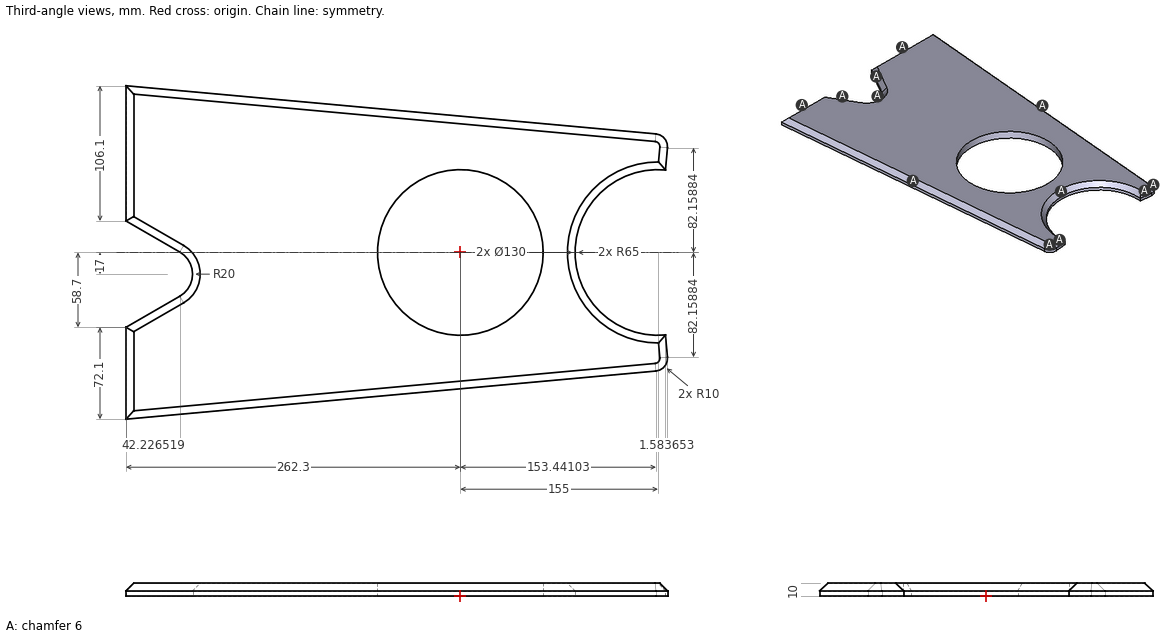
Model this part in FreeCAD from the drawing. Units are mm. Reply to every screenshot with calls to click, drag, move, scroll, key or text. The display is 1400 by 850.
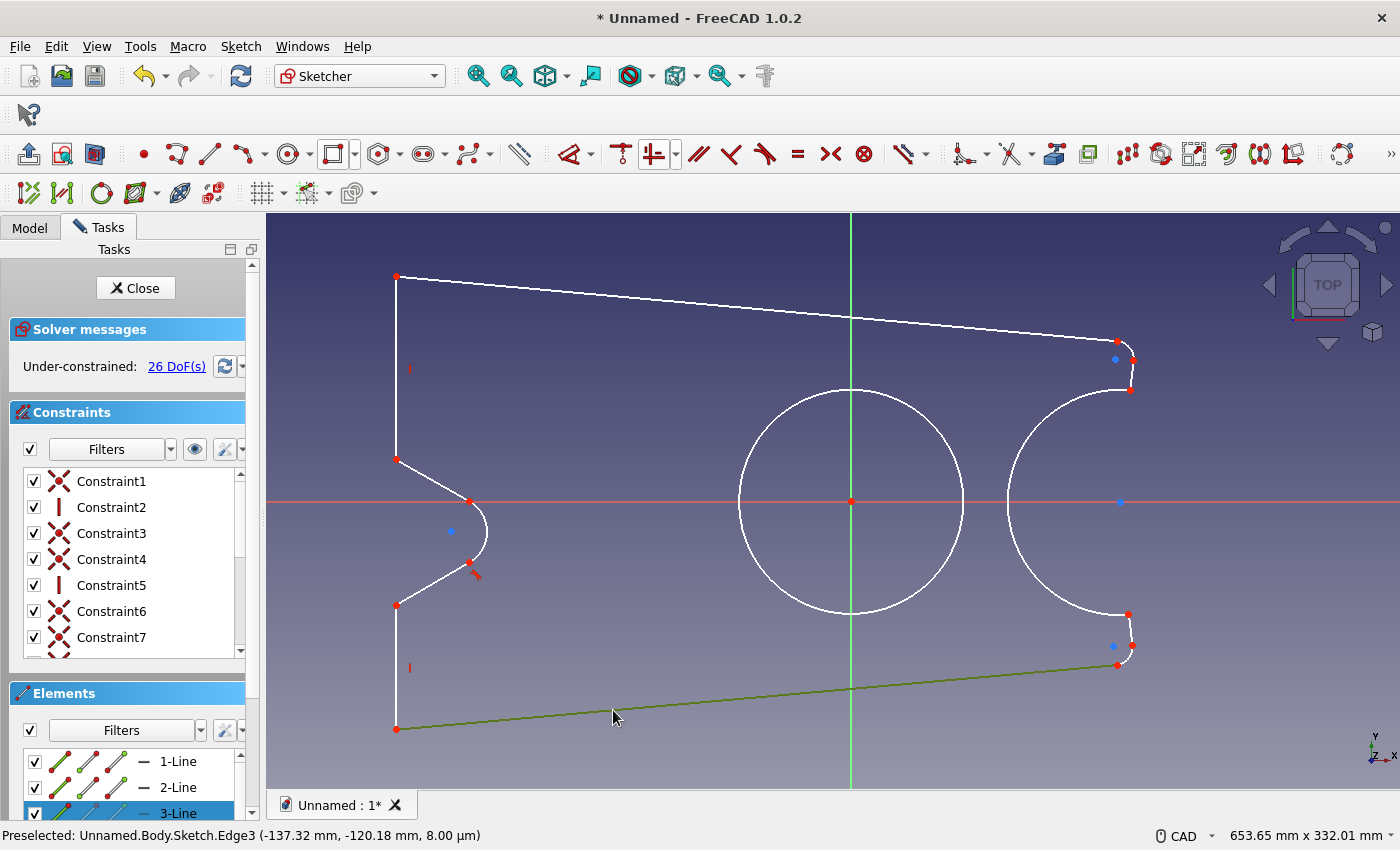
click(1129, 658)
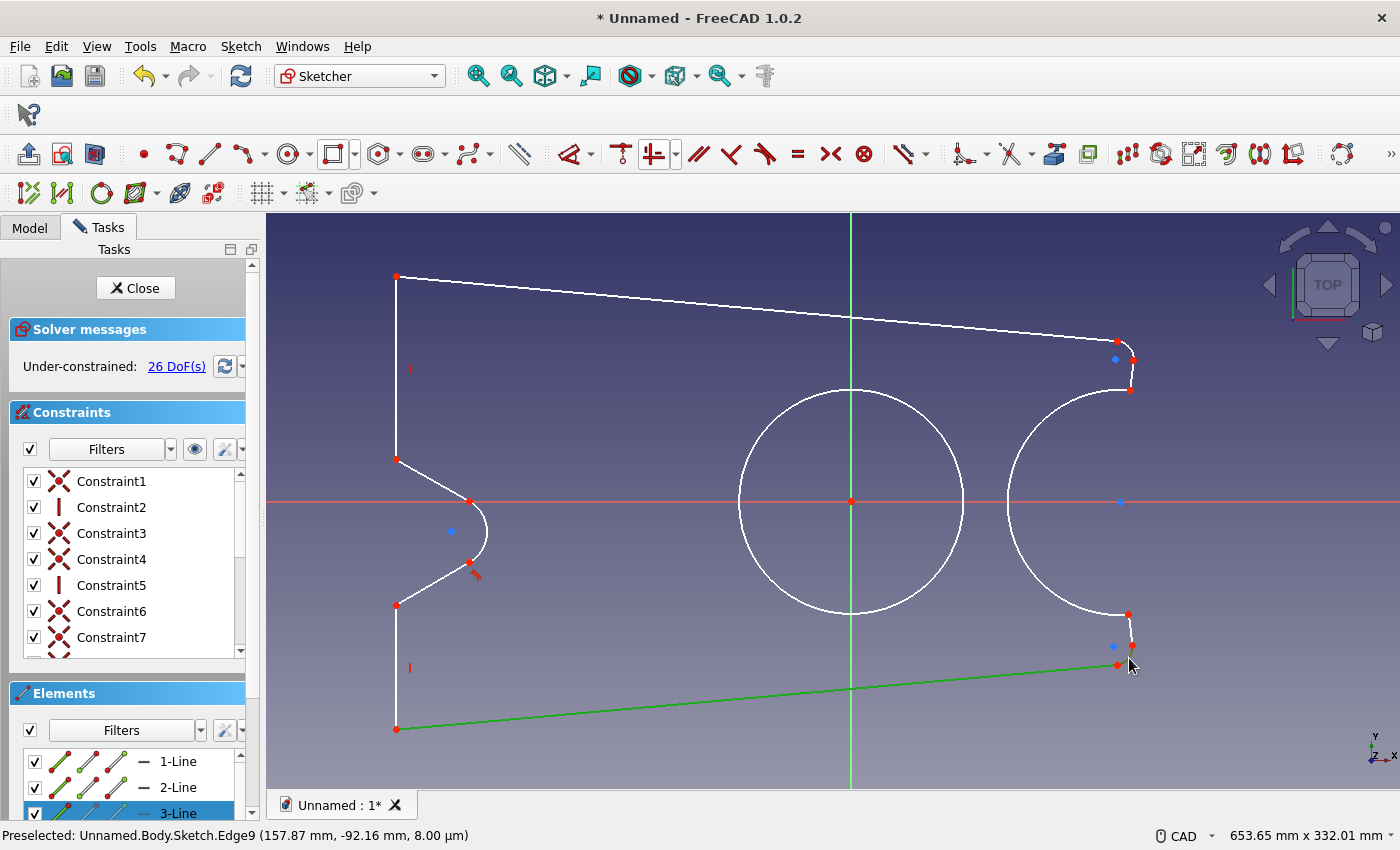
click(765, 154)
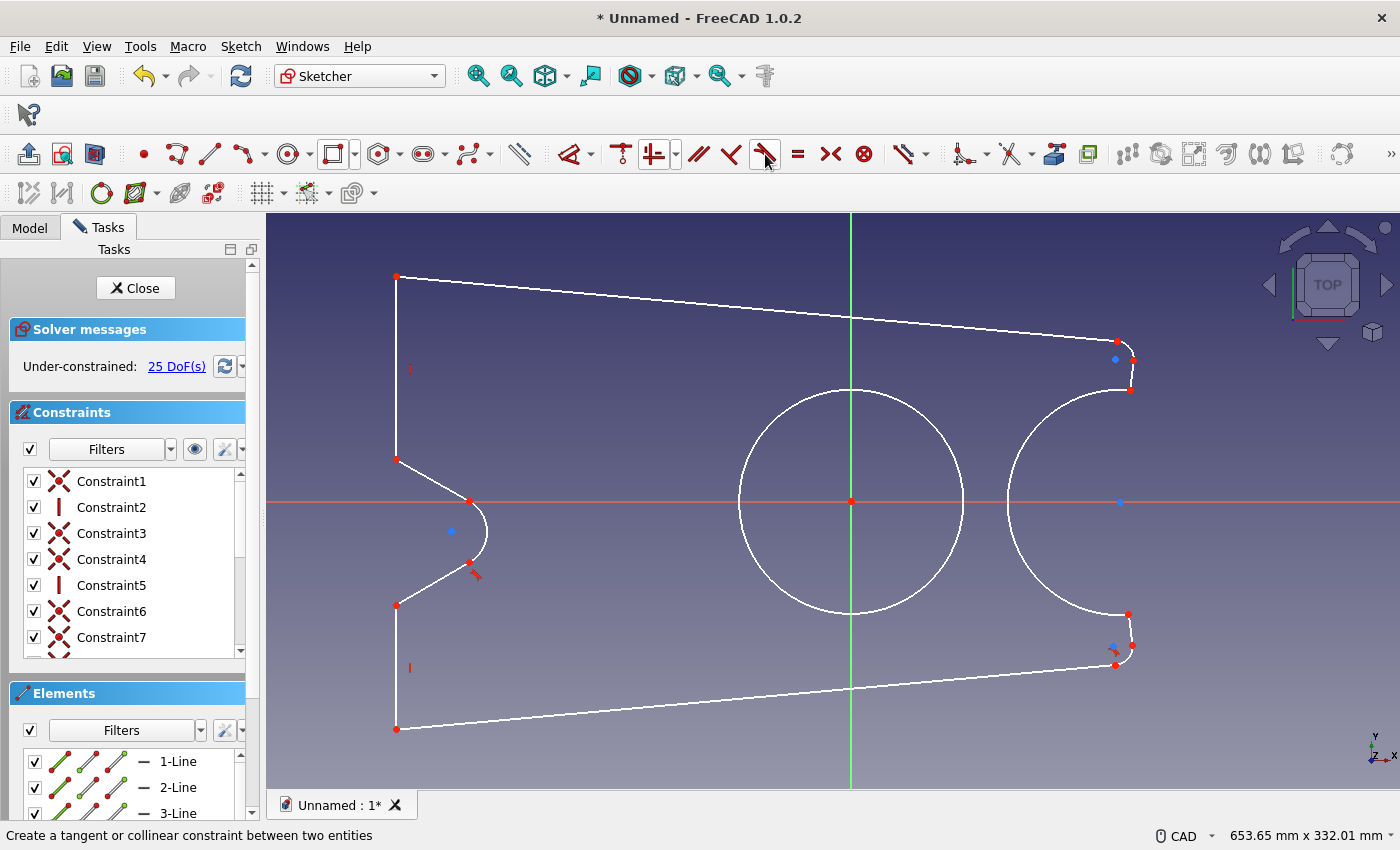
scroll(1131, 636, up, 3)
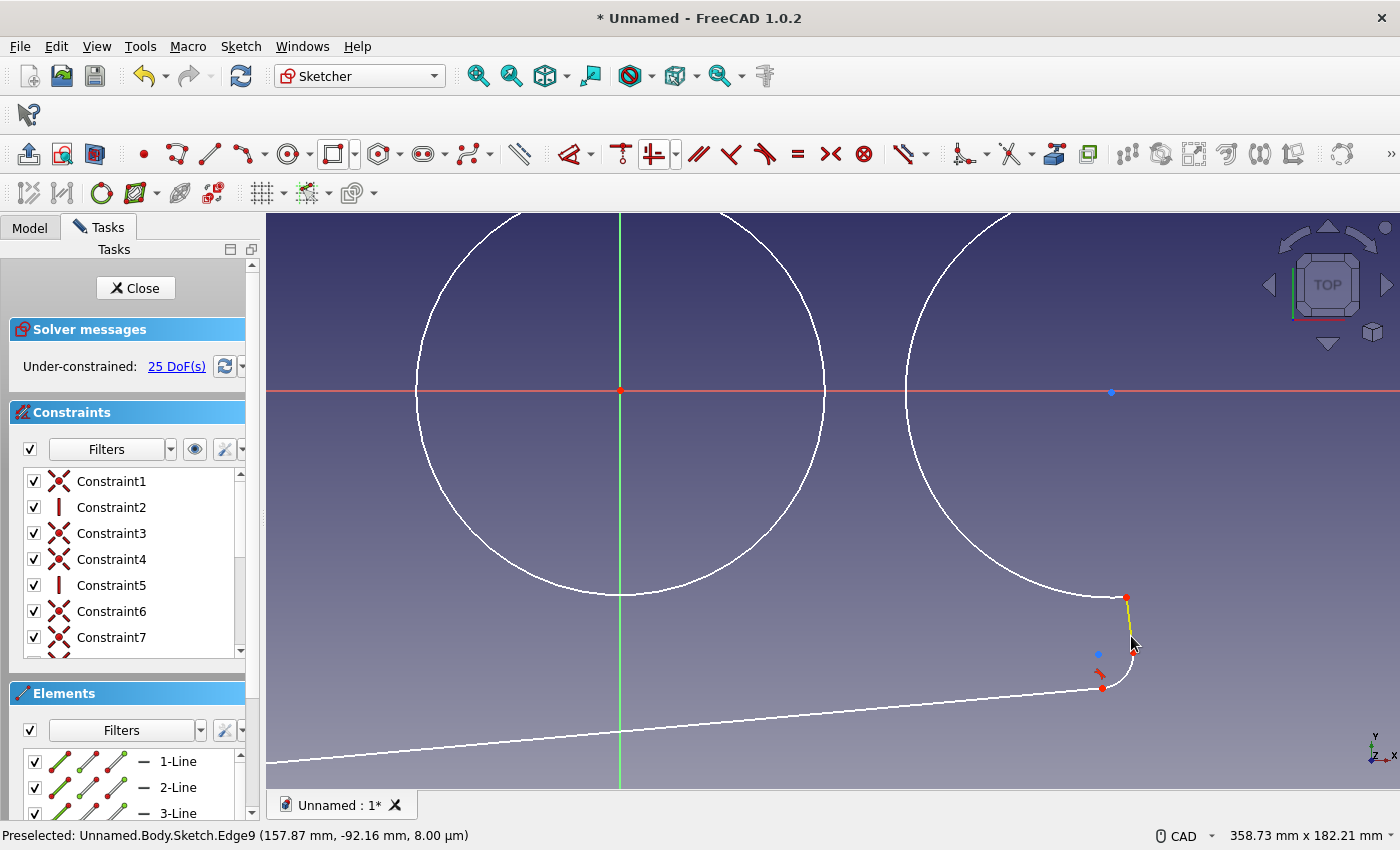
click(1131, 636)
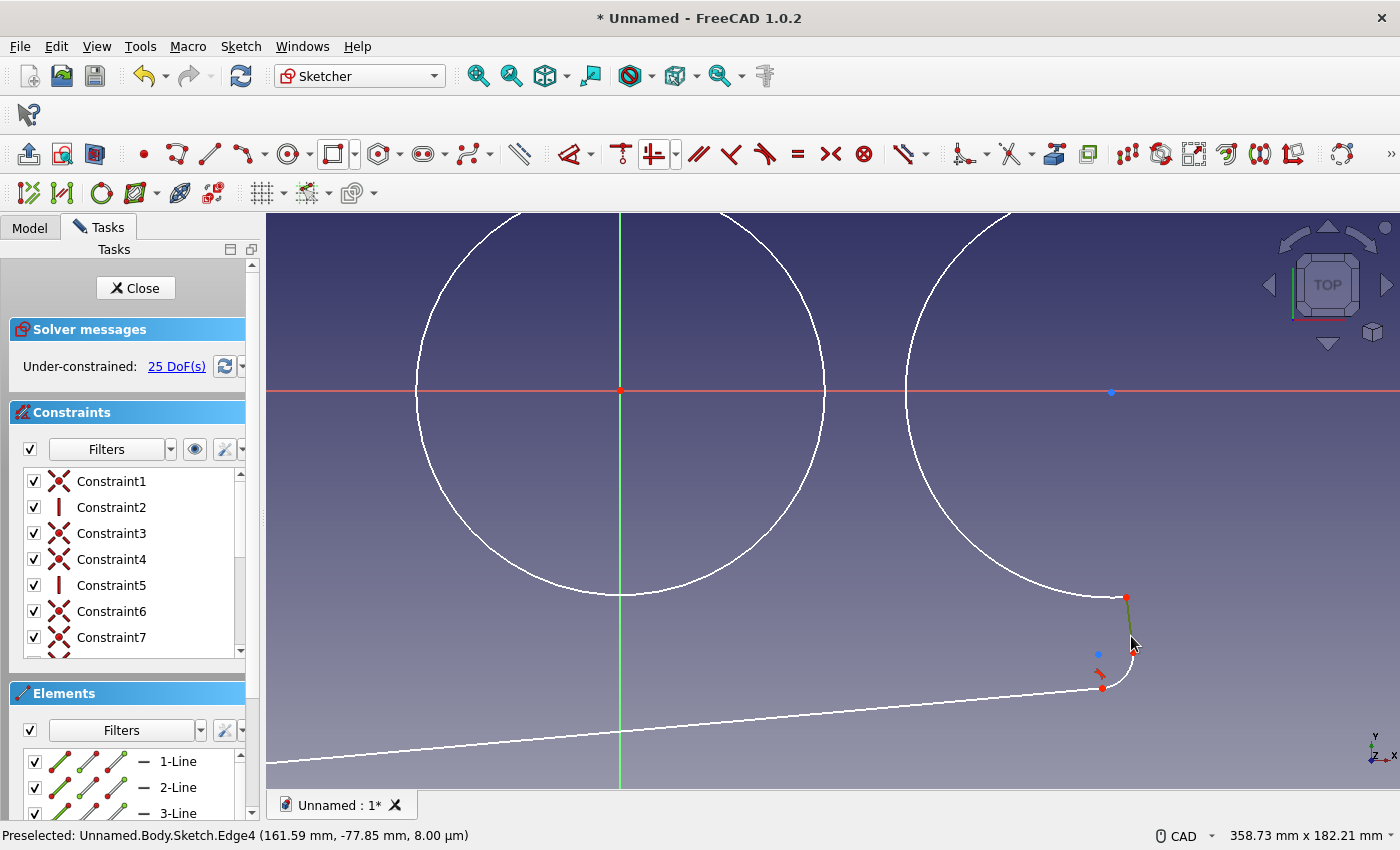
click(1117, 683)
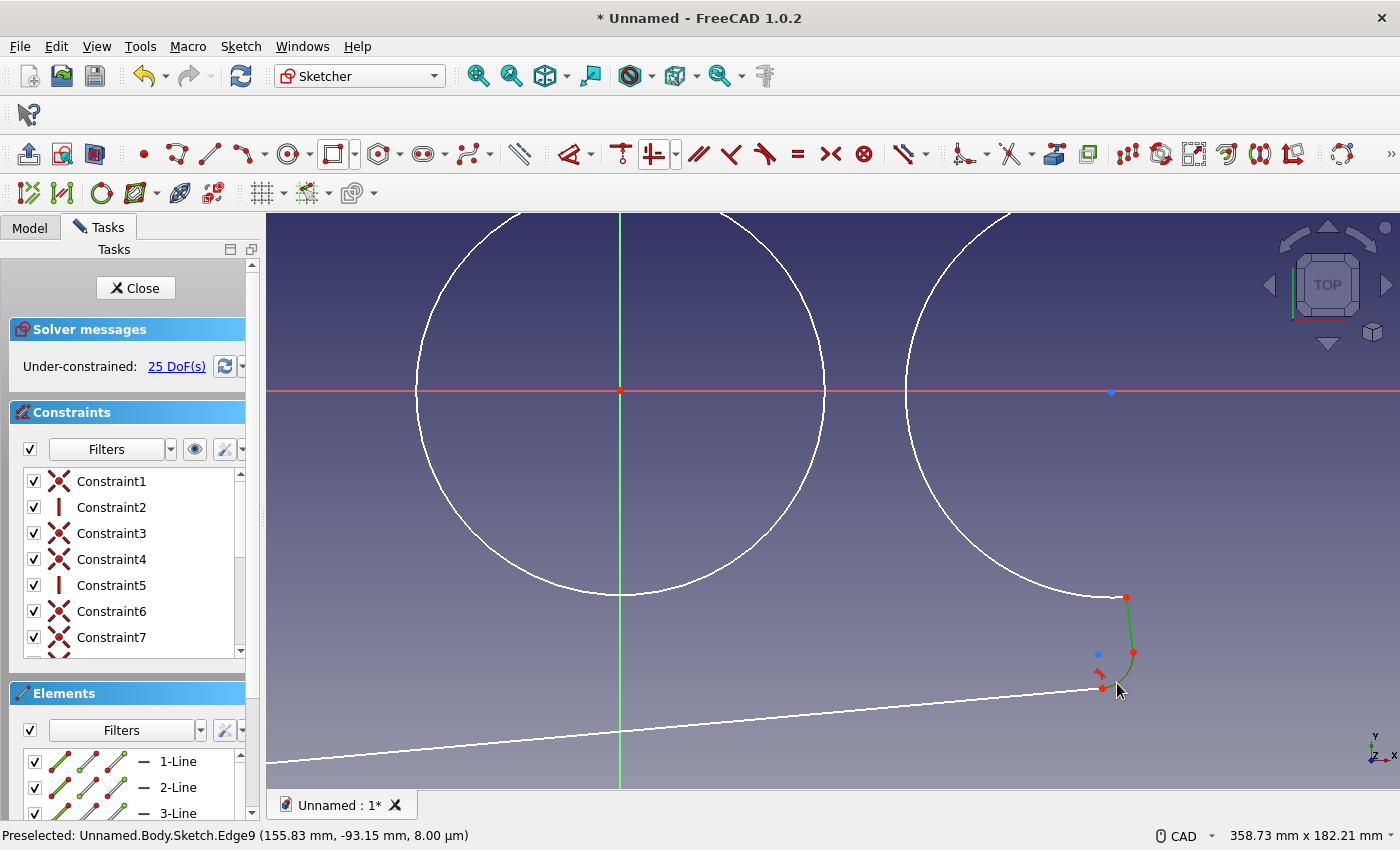
click(765, 154)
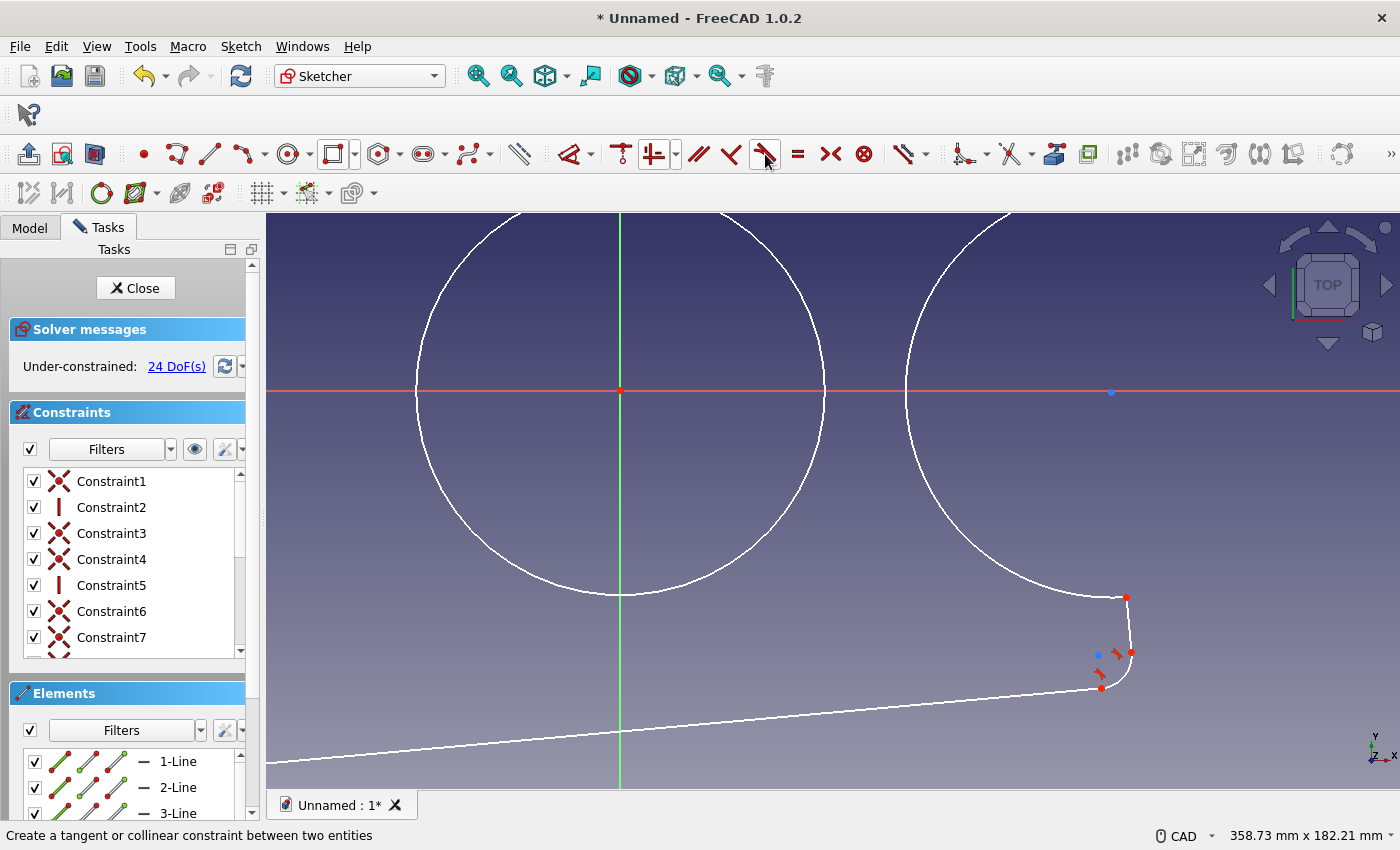
scroll(1011, 591, down, 4)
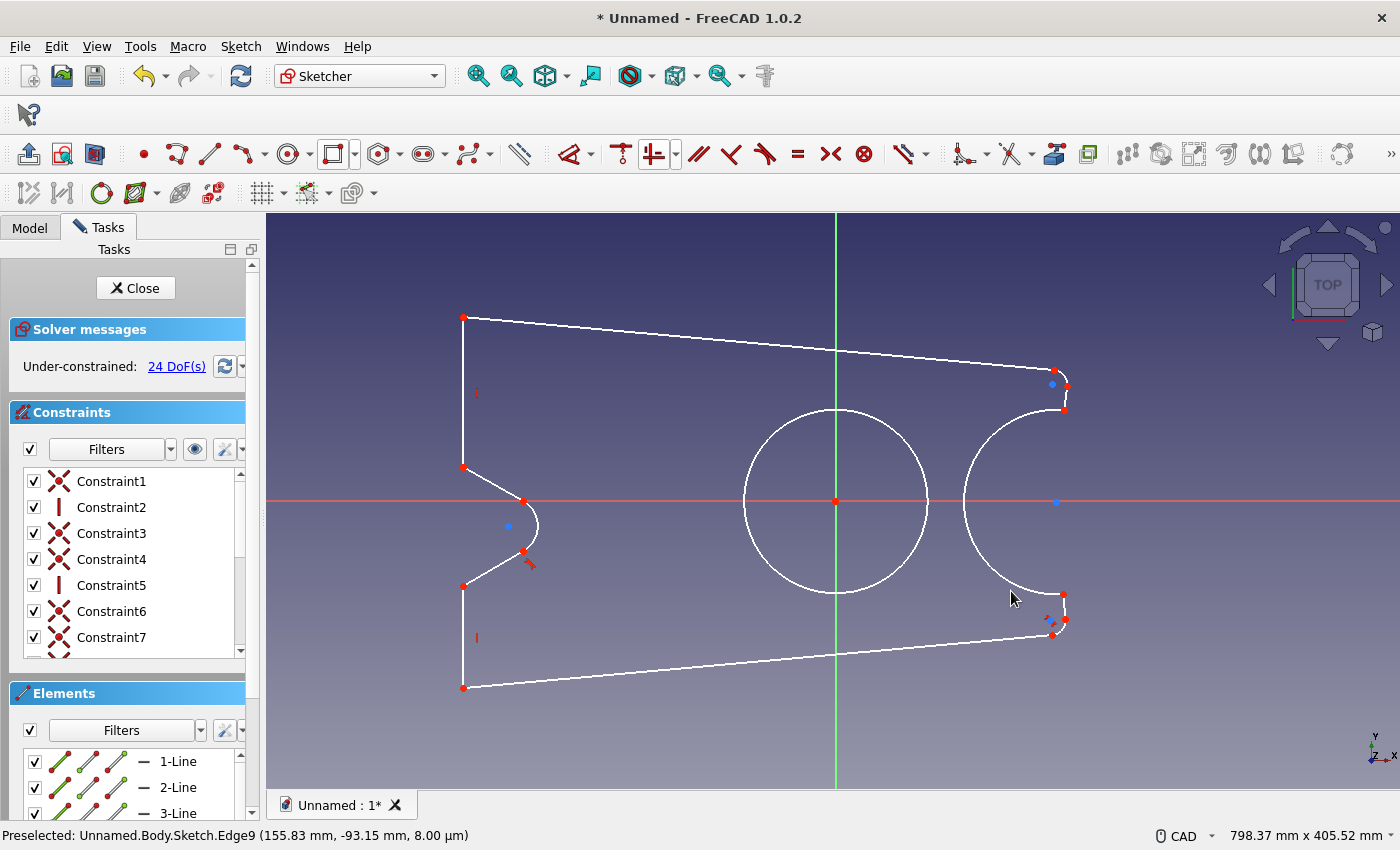
scroll(1065, 403, up, 4)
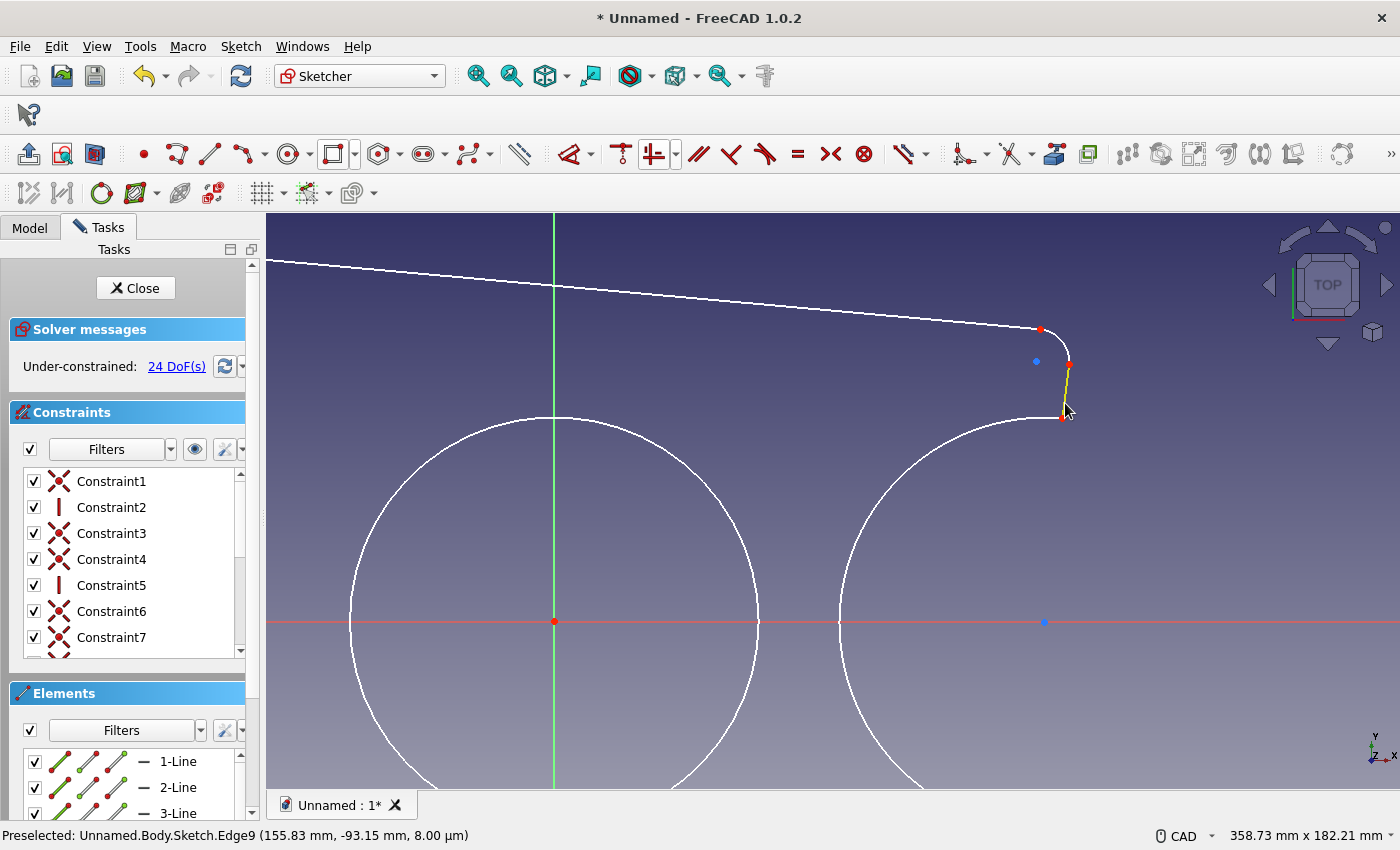
click(1064, 402)